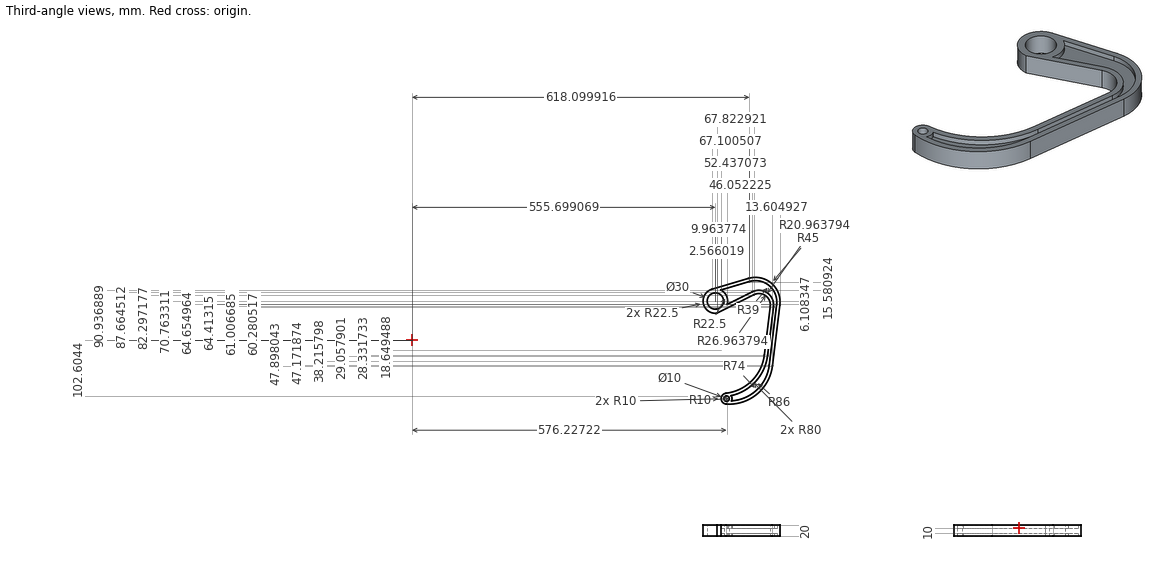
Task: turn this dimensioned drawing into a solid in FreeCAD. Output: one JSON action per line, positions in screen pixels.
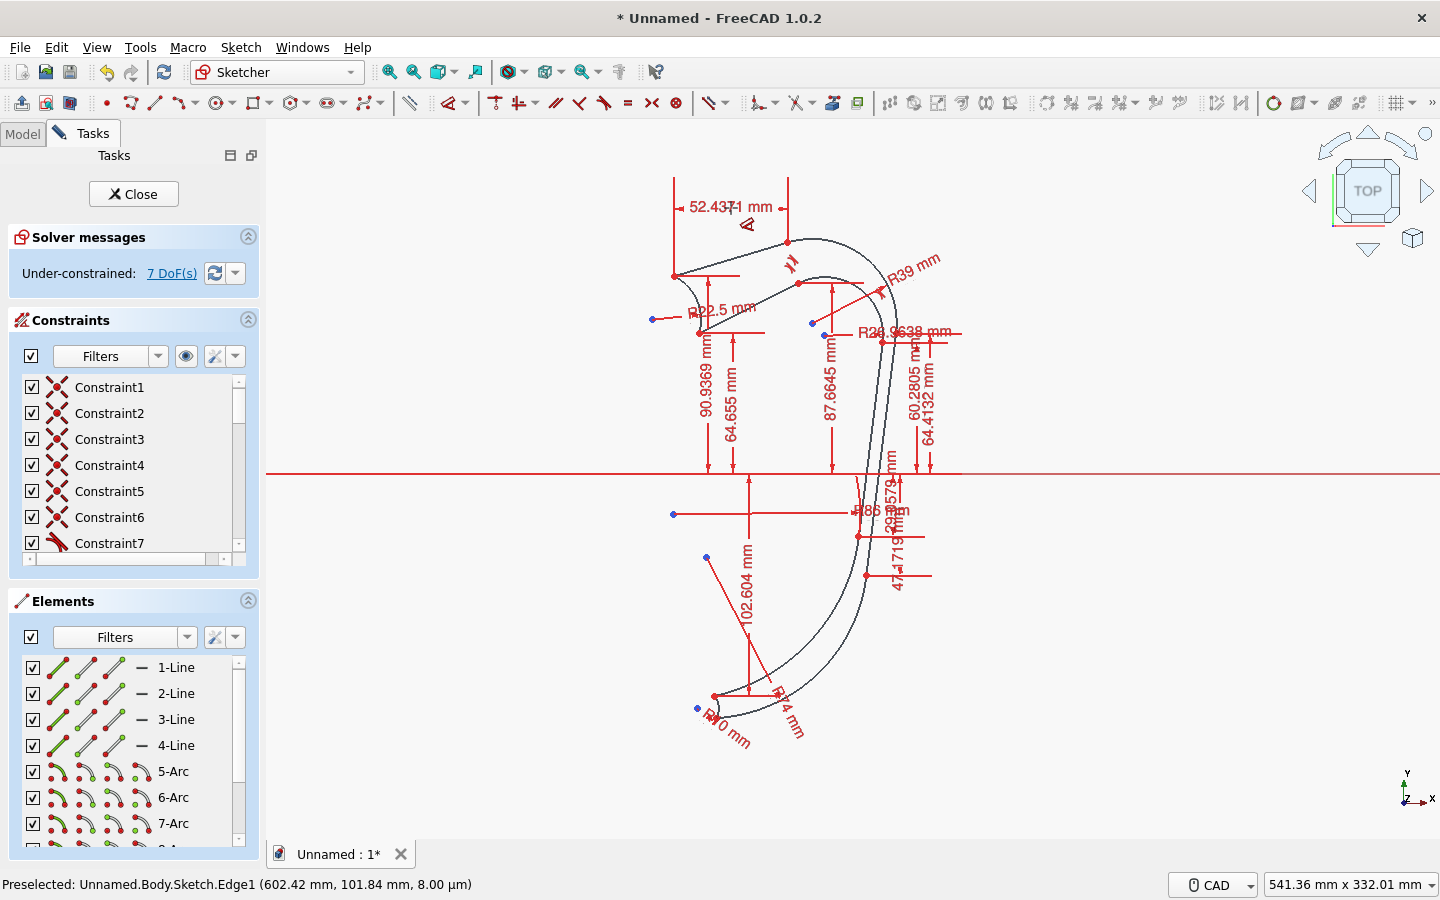
{"action": "left_click", "coordinate": [754, 253]}
{"action": "left_click", "coordinate": [640, 259]}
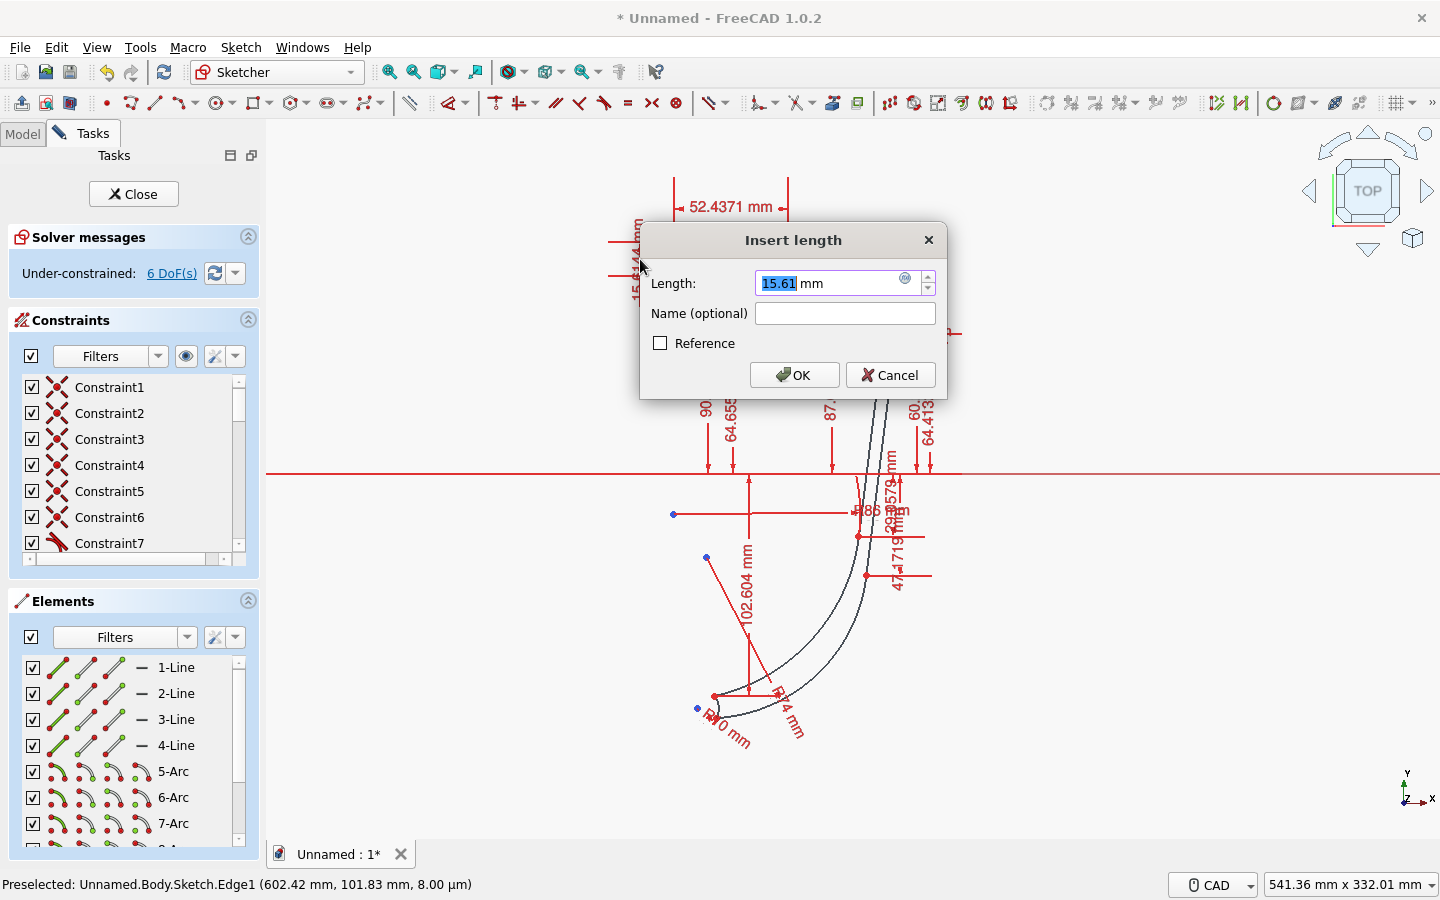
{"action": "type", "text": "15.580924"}
{"action": "key", "text": "Return"}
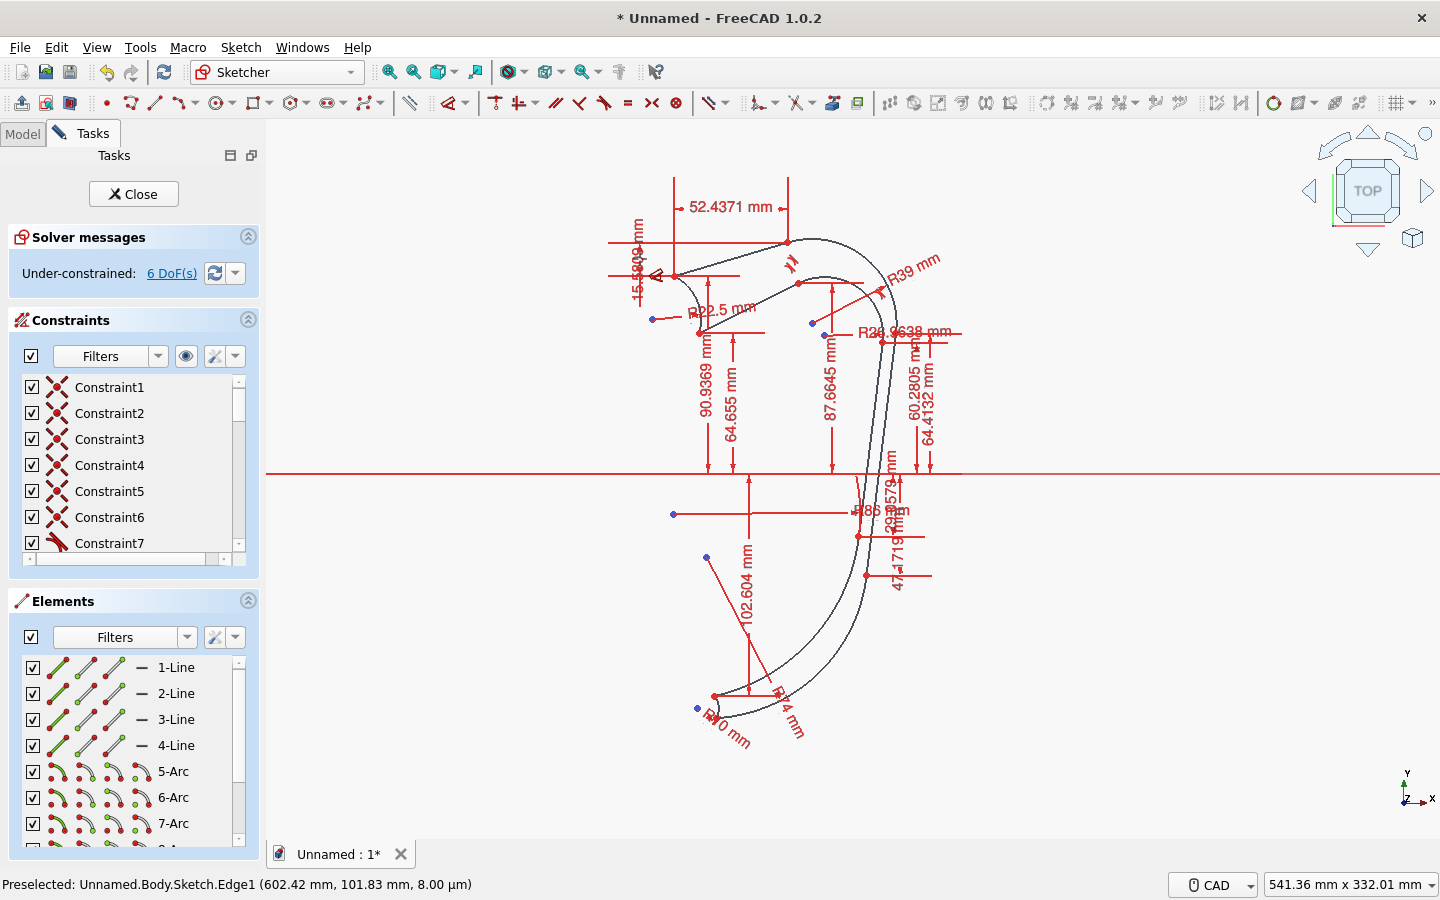
{"action": "left_click", "coordinate": [729, 318]}
{"action": "left_click", "coordinate": [714, 249]}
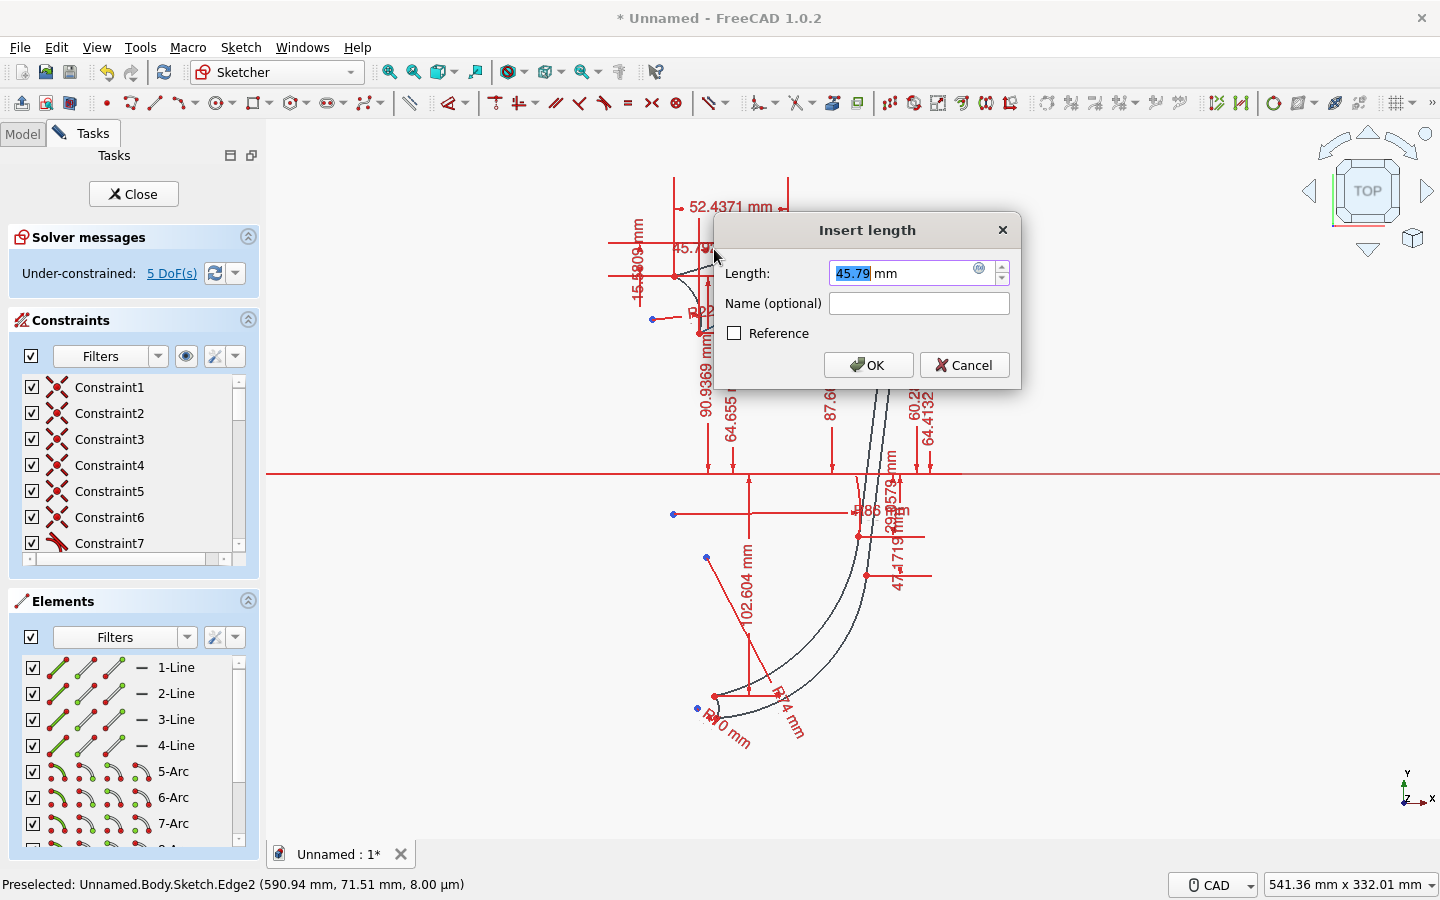
{"action": "type", "text": "46.052225"}
{"action": "key", "text": "Return"}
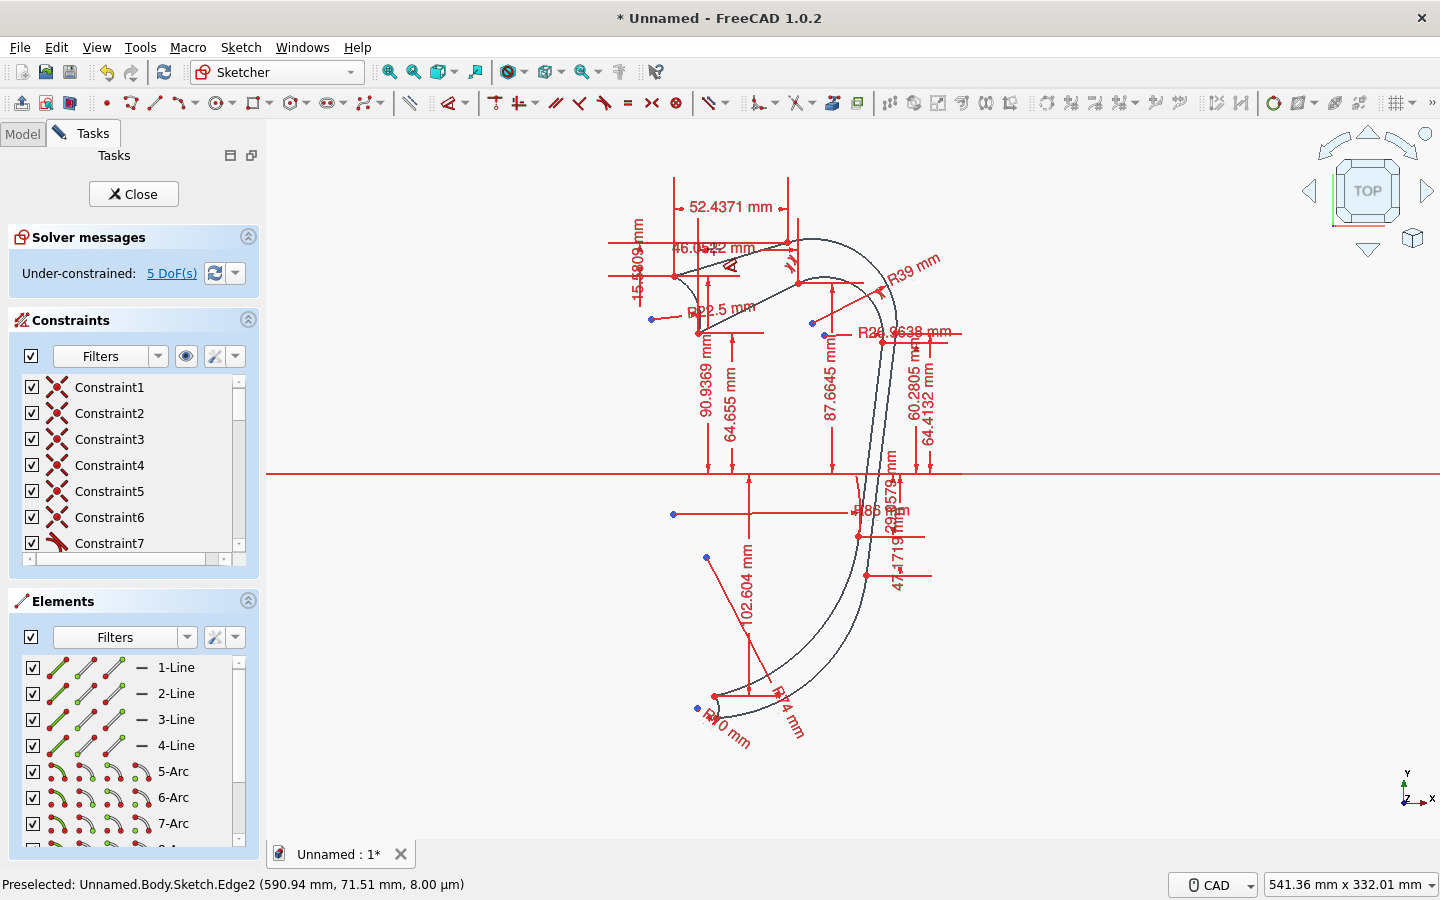
{"action": "left_click", "coordinate": [652, 320]}
{"action": "left_click", "coordinate": [686, 432]}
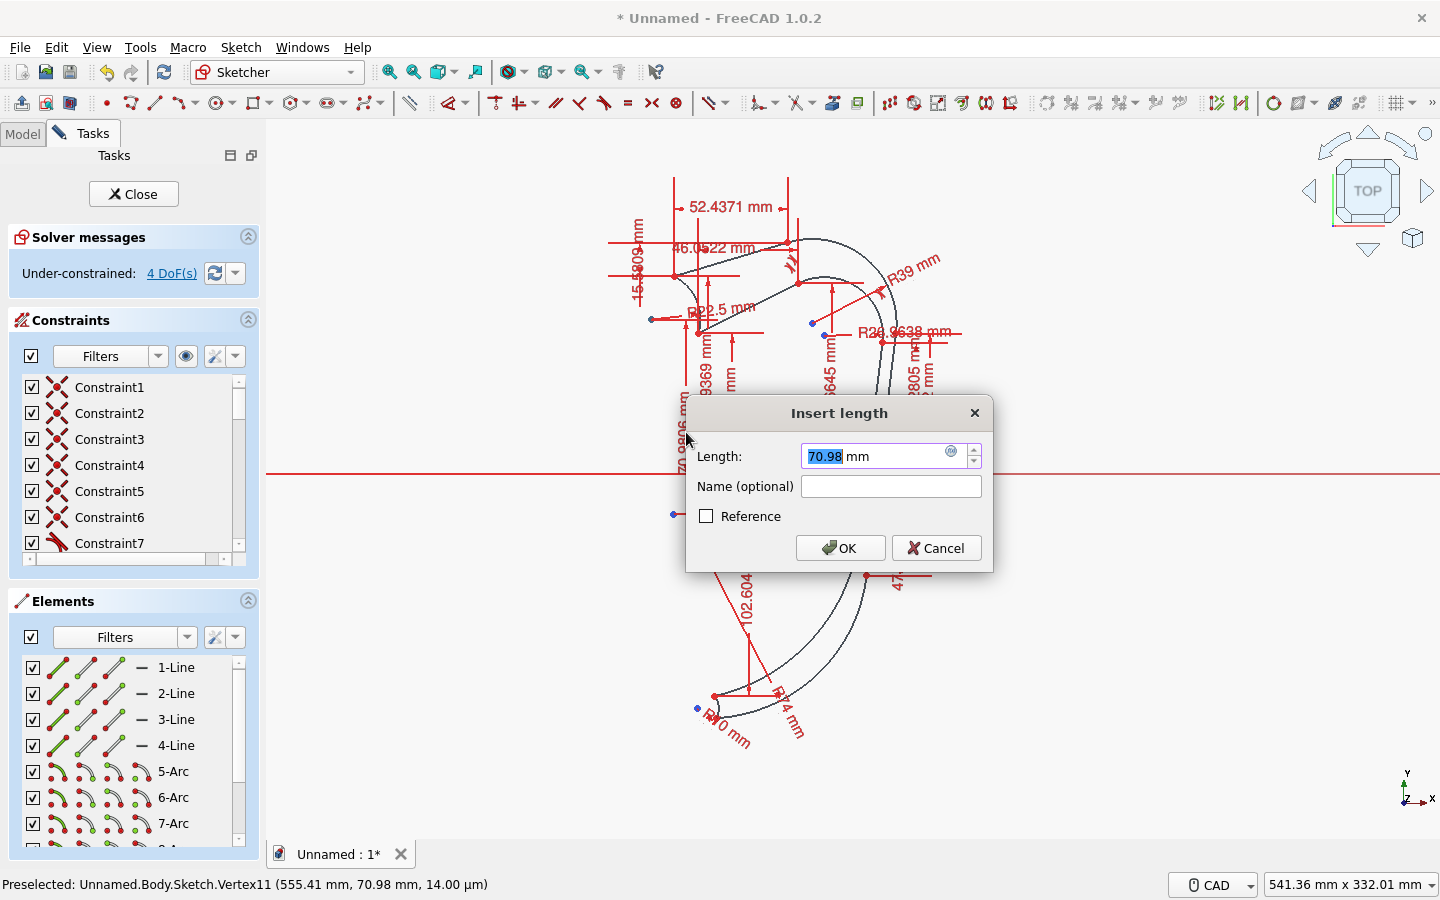
{"action": "type", "text": "70.763311"}
{"action": "key", "text": "Return"}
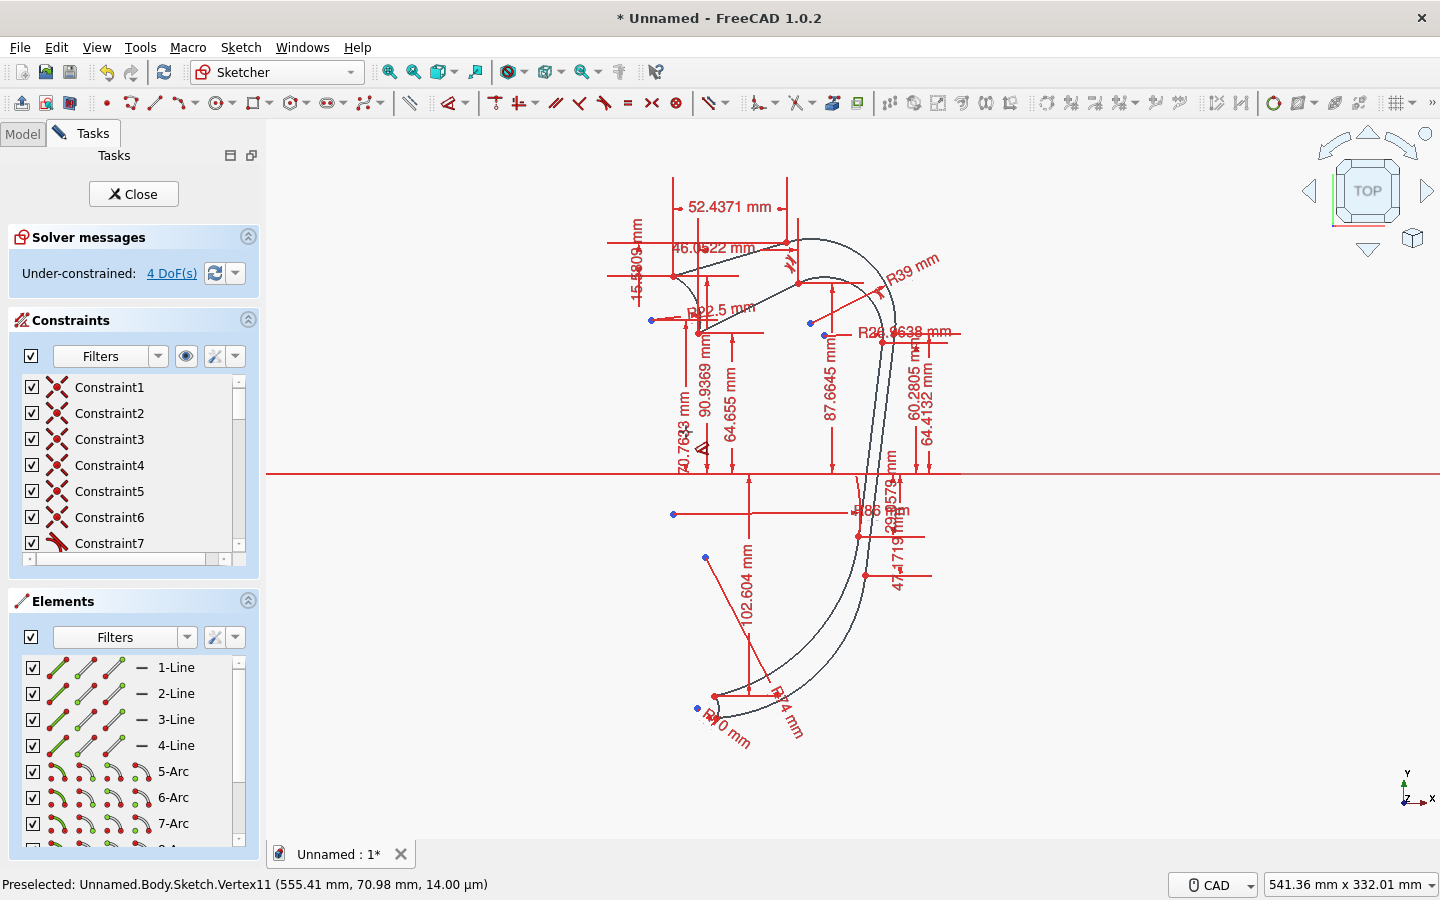
{"action": "left_click", "coordinate": [674, 514]}
{"action": "left_click", "coordinate": [708, 494]}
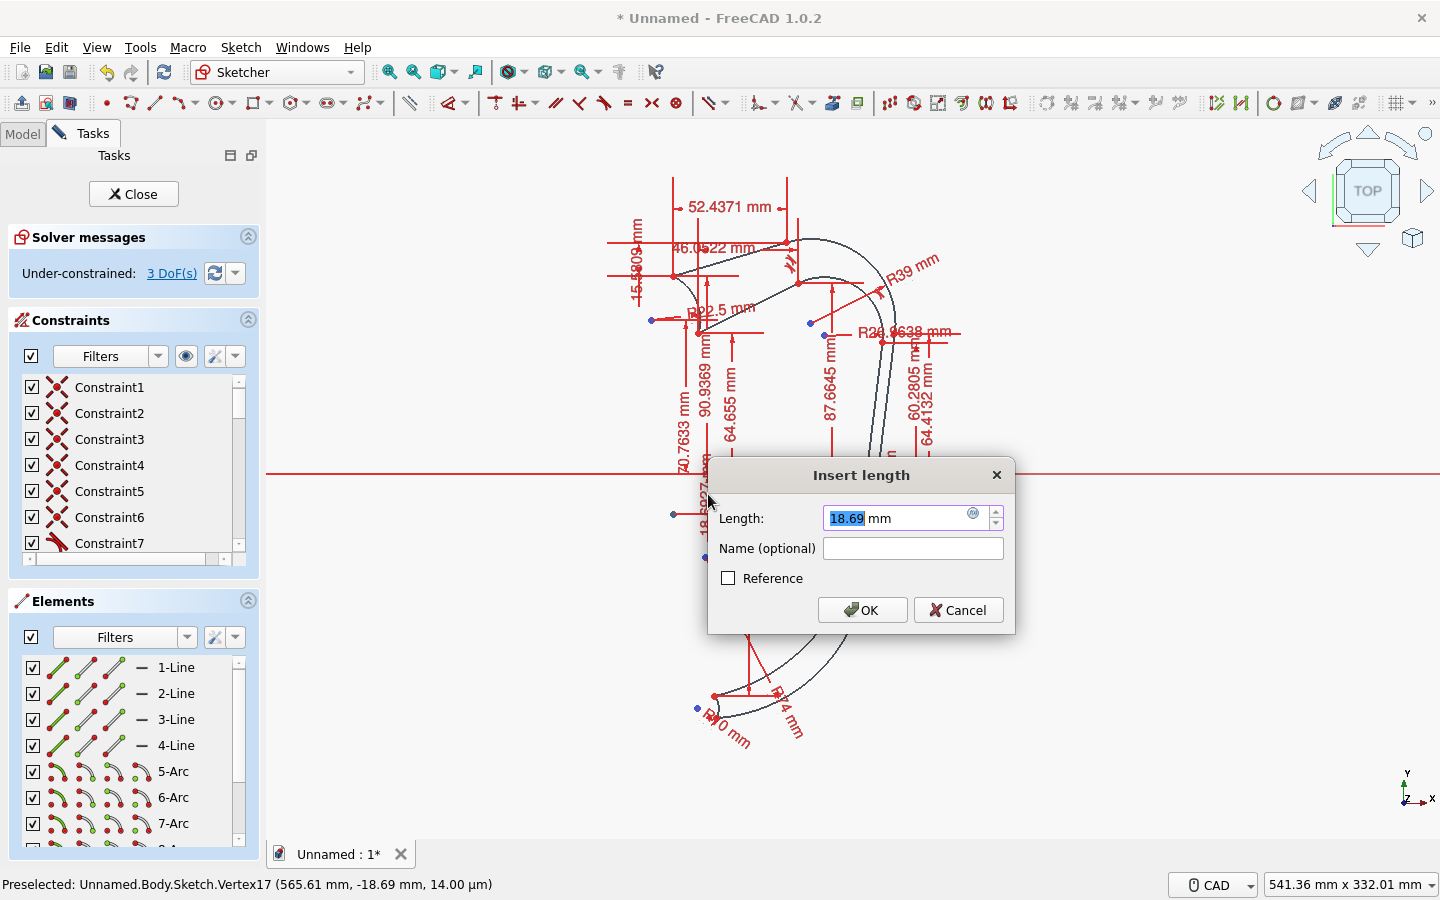
{"action": "type", "text": "18.649488"}
{"action": "key", "text": "Return"}